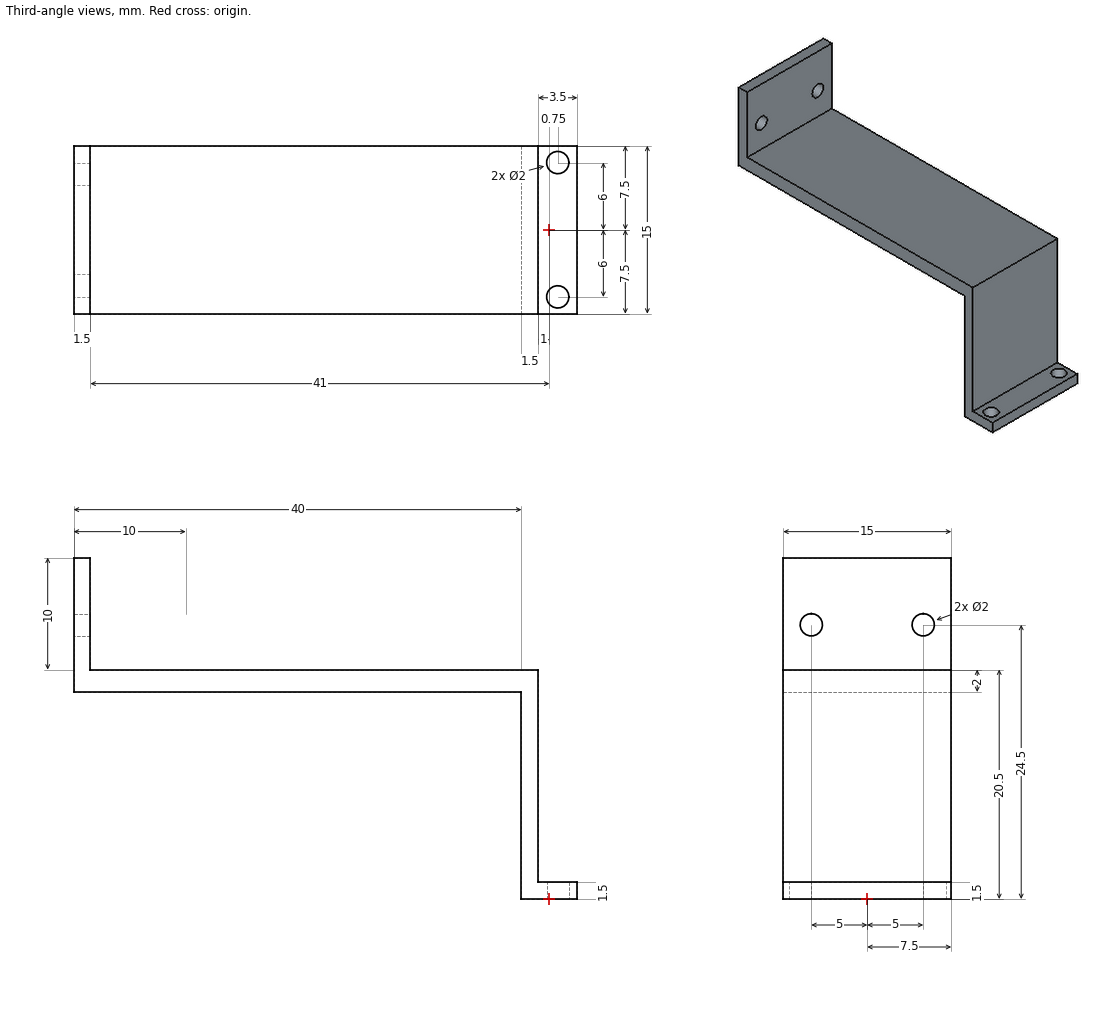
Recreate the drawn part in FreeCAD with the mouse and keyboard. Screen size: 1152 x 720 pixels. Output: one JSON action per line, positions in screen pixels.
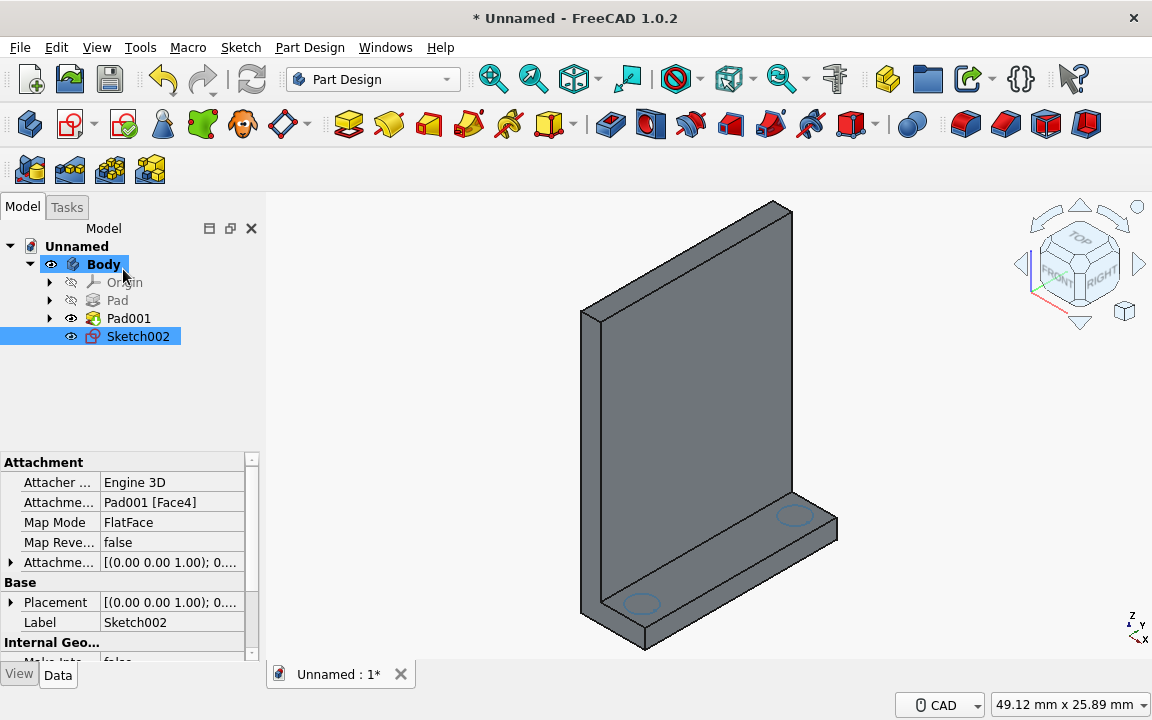
{"action": "left_click", "coordinate": [612, 124]}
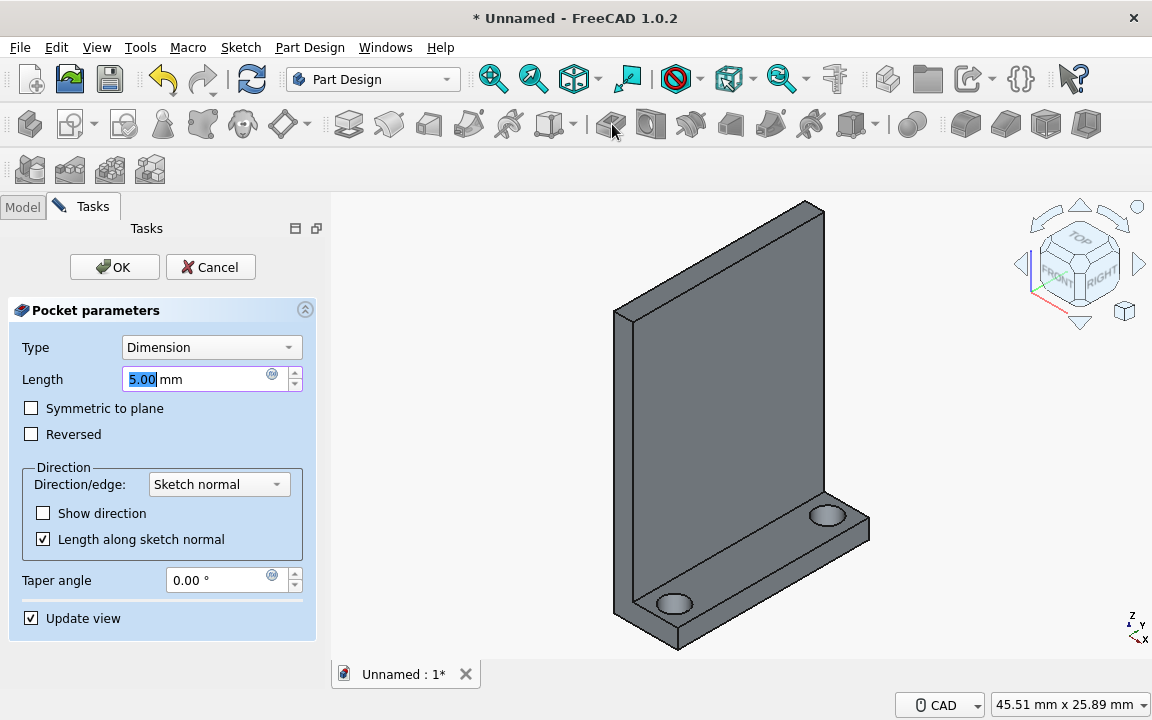
{"action": "type", "text": "1.5"}
{"action": "key", "text": "Tab"}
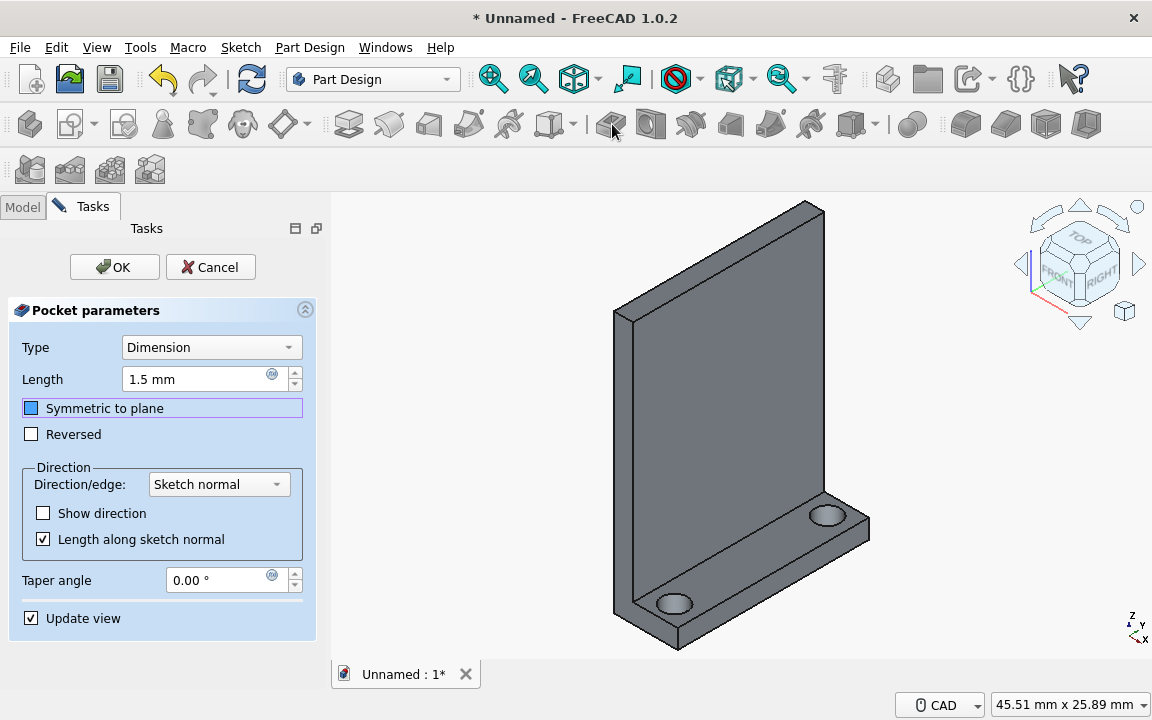
{"action": "left_click", "coordinate": [115, 267]}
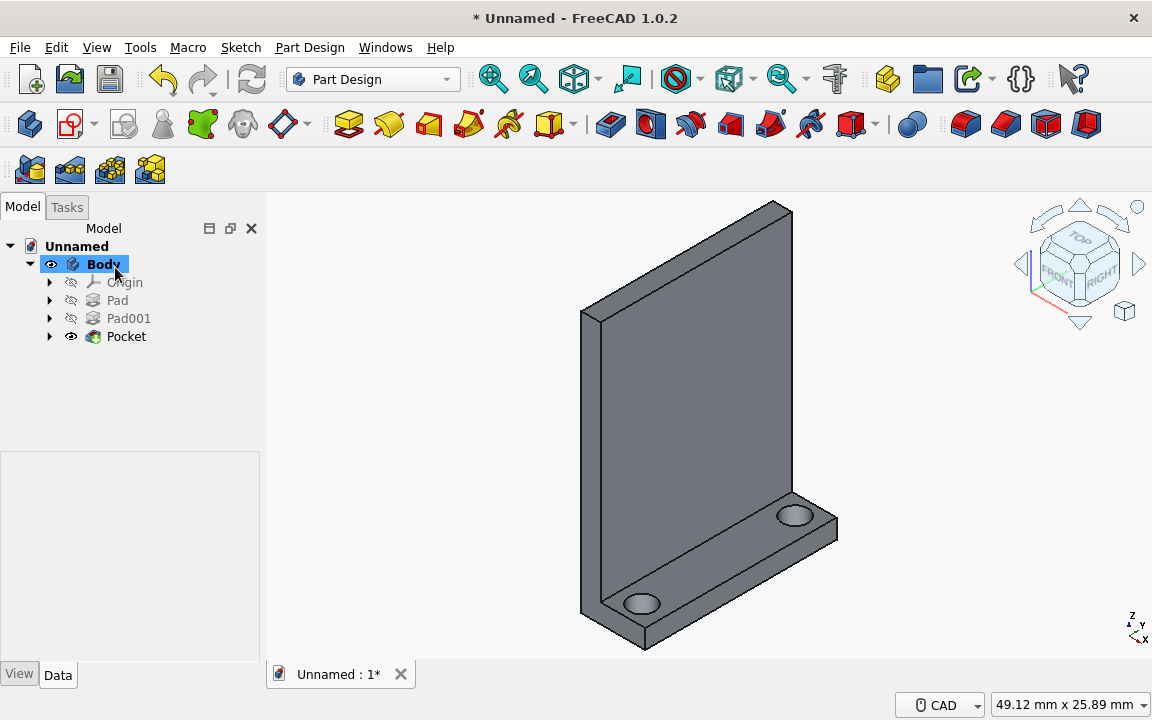
{"action": "key", "text": "6"}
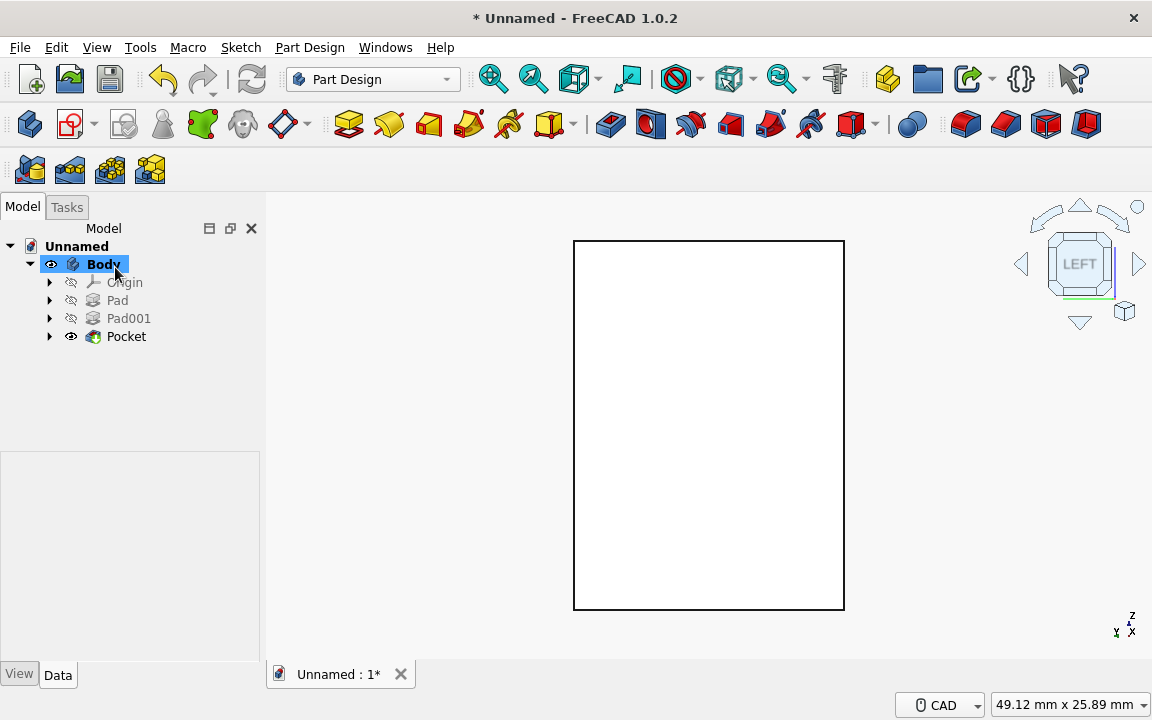
{"action": "left_click", "coordinate": [709, 424]}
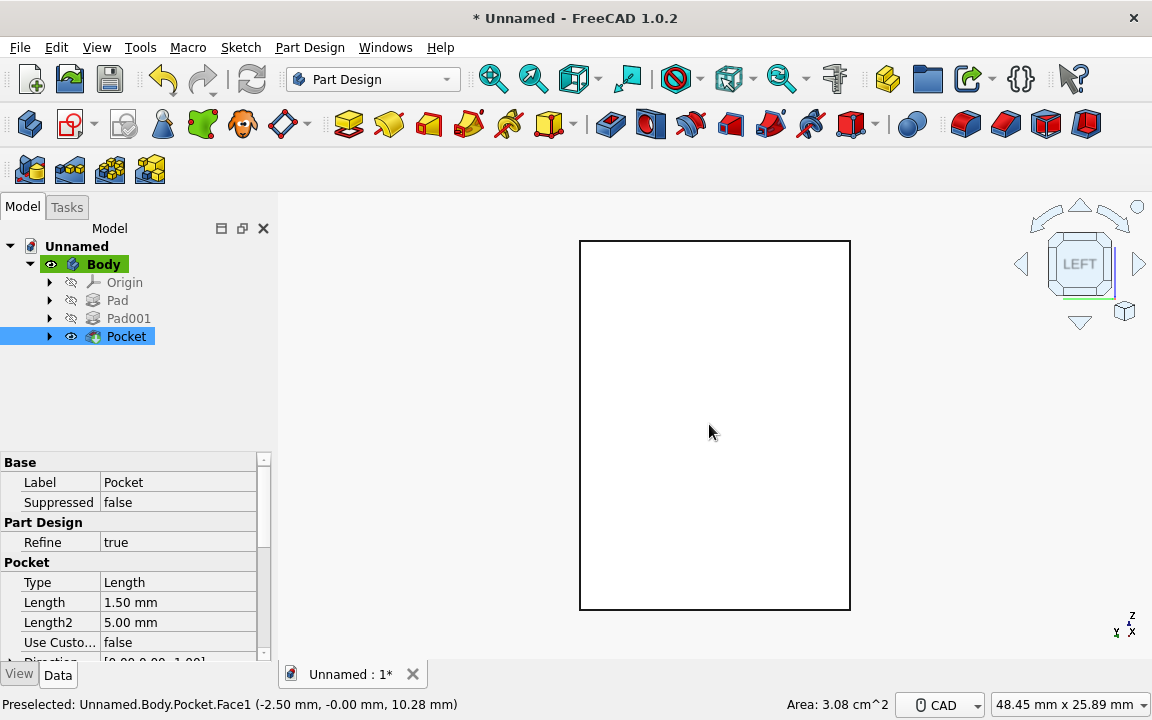
{"action": "left_click", "coordinate": [70, 124]}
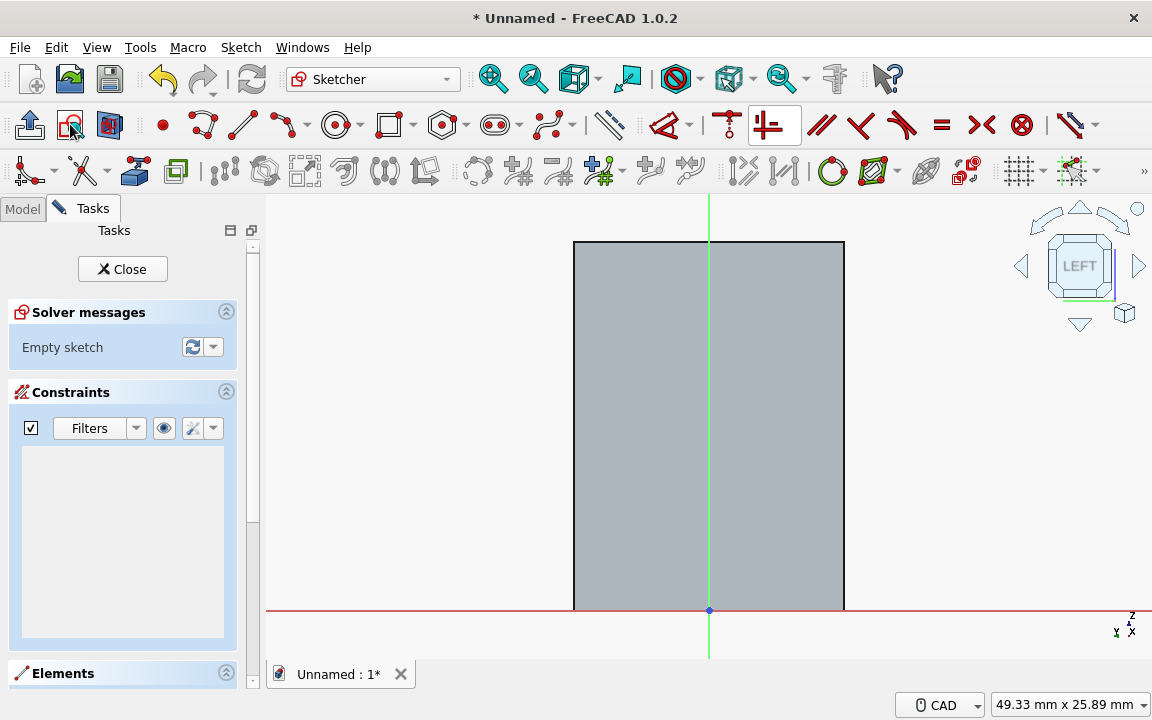
{"action": "scroll", "coordinate": [331, 427], "scroll_direction": "down", "scroll_amount": 1}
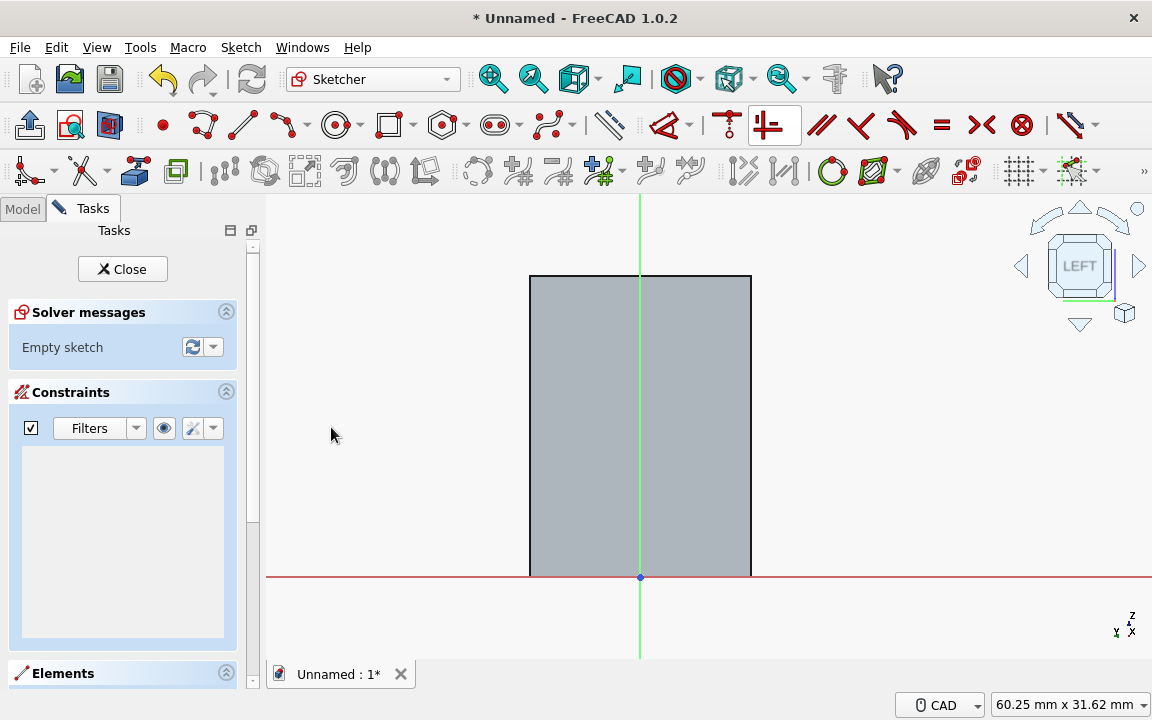
{"action": "left_click", "coordinate": [390, 126]}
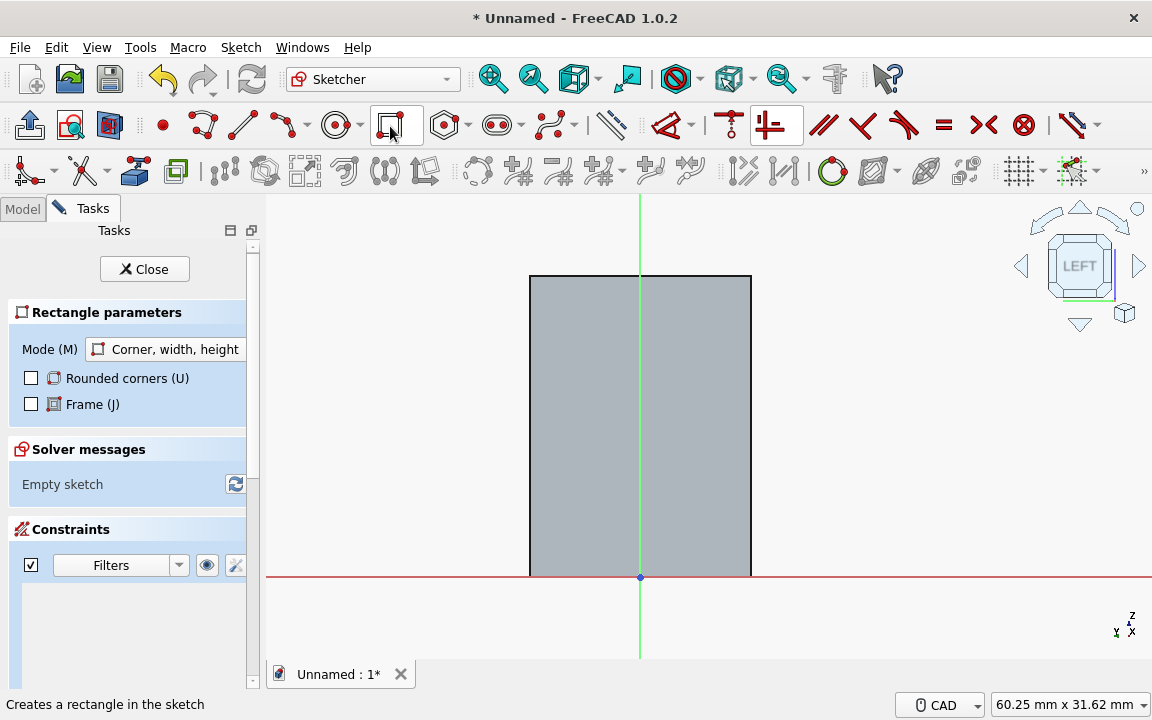
{"action": "left_click", "coordinate": [530, 276]}
{"action": "left_click", "coordinate": [751, 305]}
{"action": "key", "text": "Escape"}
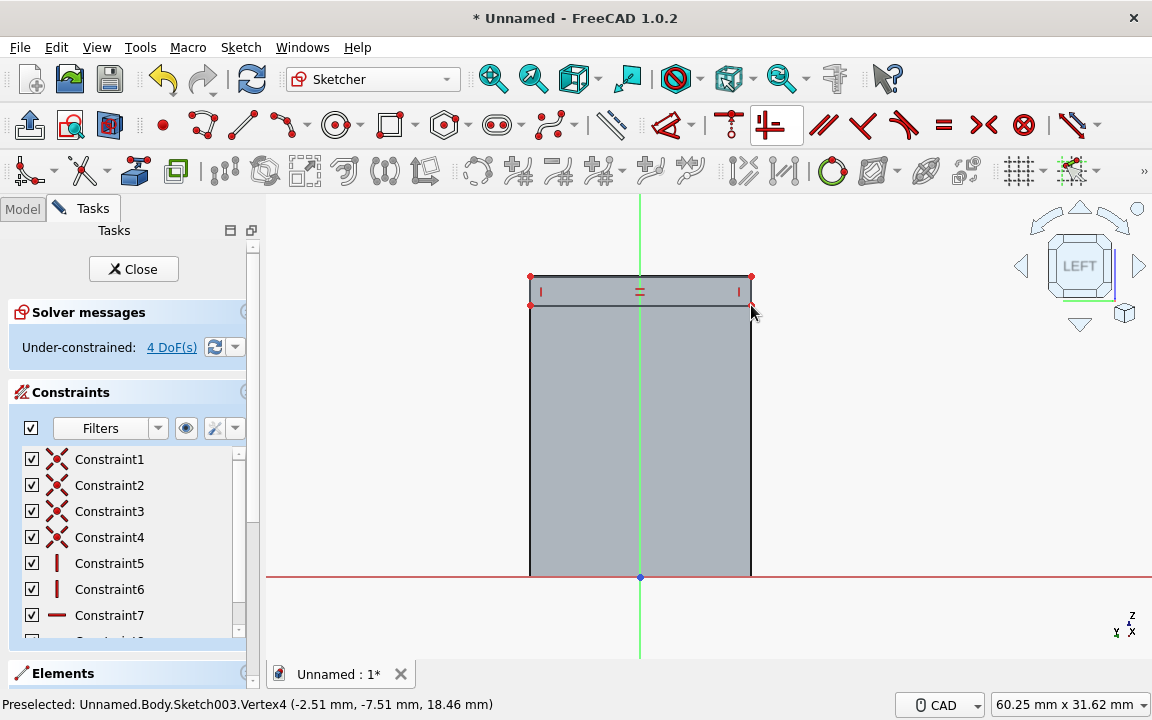
{"action": "left_click", "coordinate": [666, 126]}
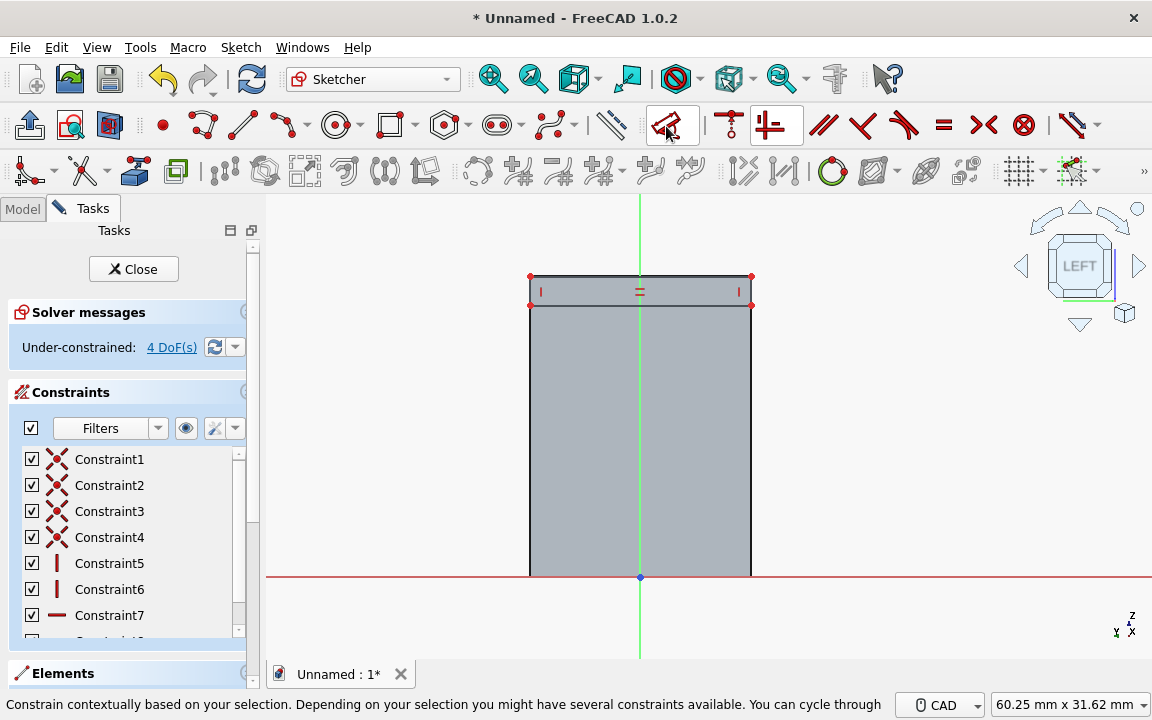
{"action": "scroll", "coordinate": [530, 289], "scroll_direction": "up", "scroll_amount": 2}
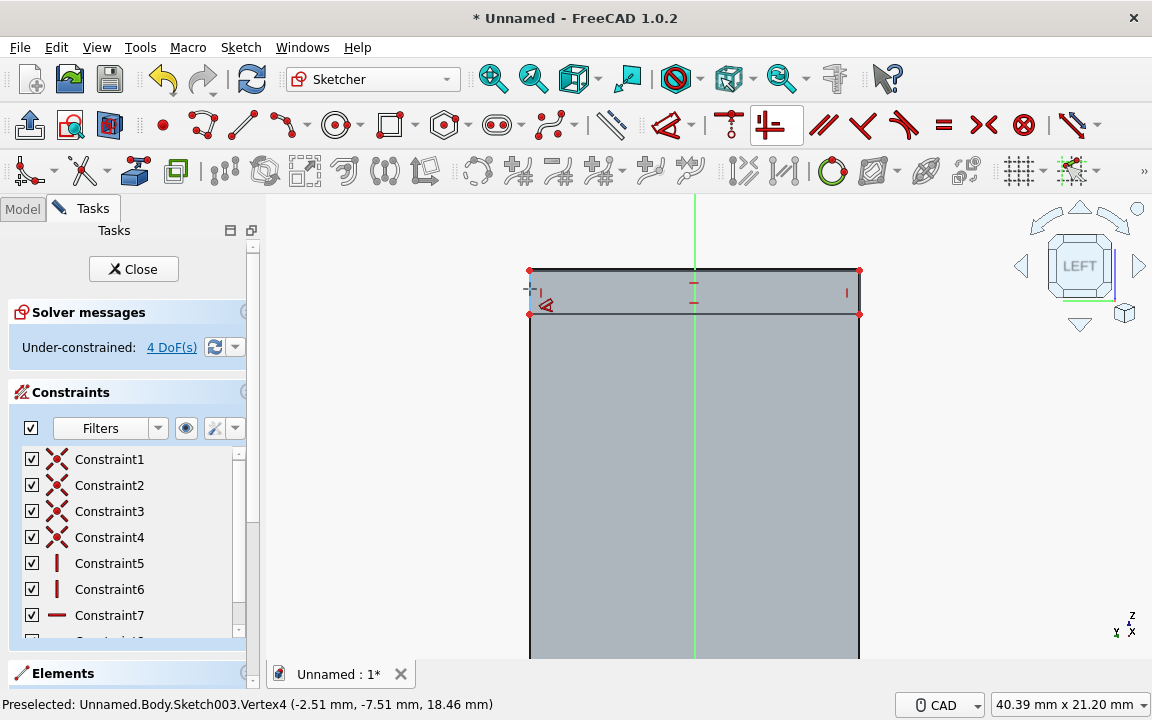
{"action": "left_click", "coordinate": [530, 288]}
{"action": "left_click", "coordinate": [496, 293]}